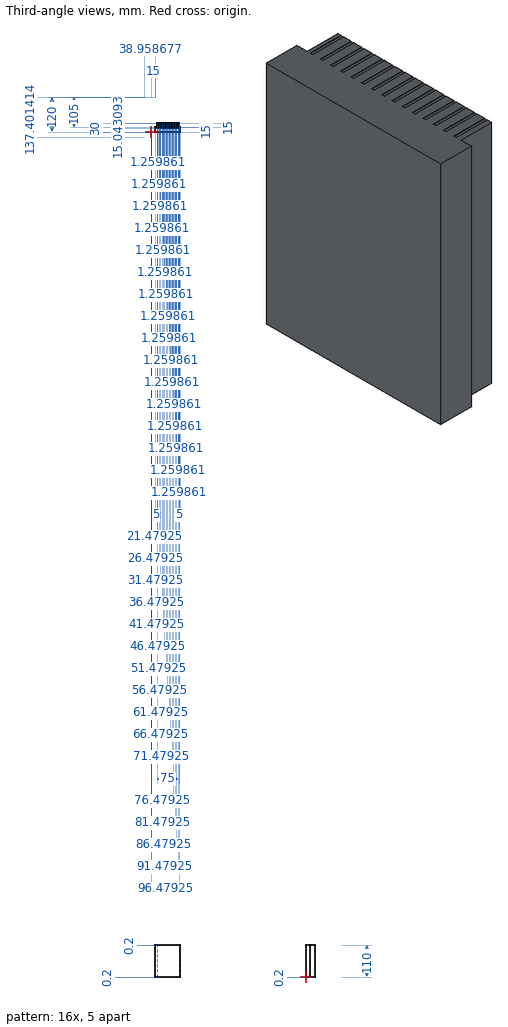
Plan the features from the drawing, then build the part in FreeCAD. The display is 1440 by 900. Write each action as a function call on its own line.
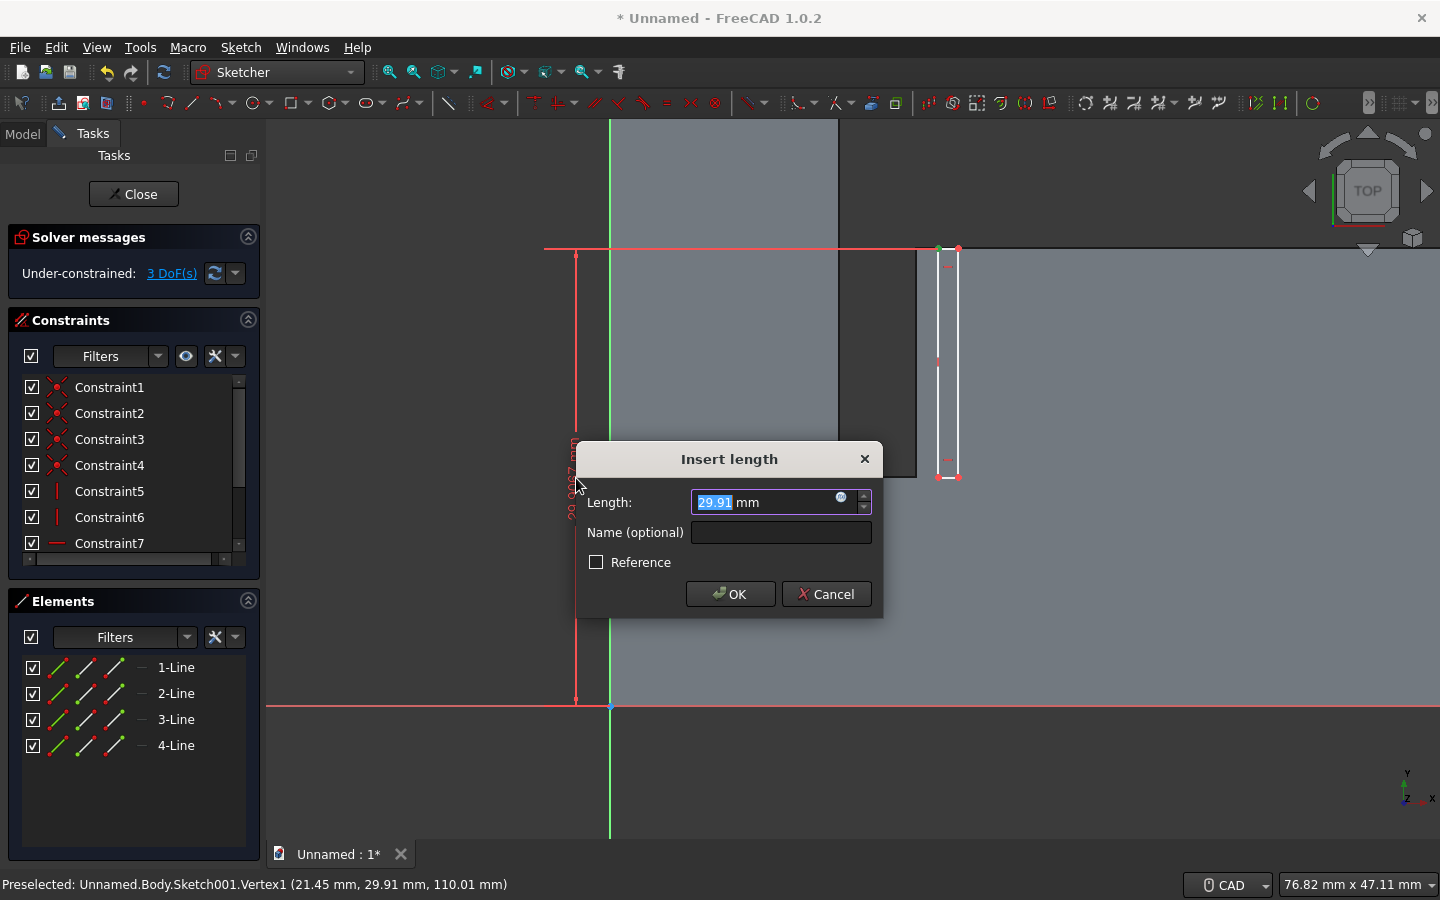
text(30)
key(Return)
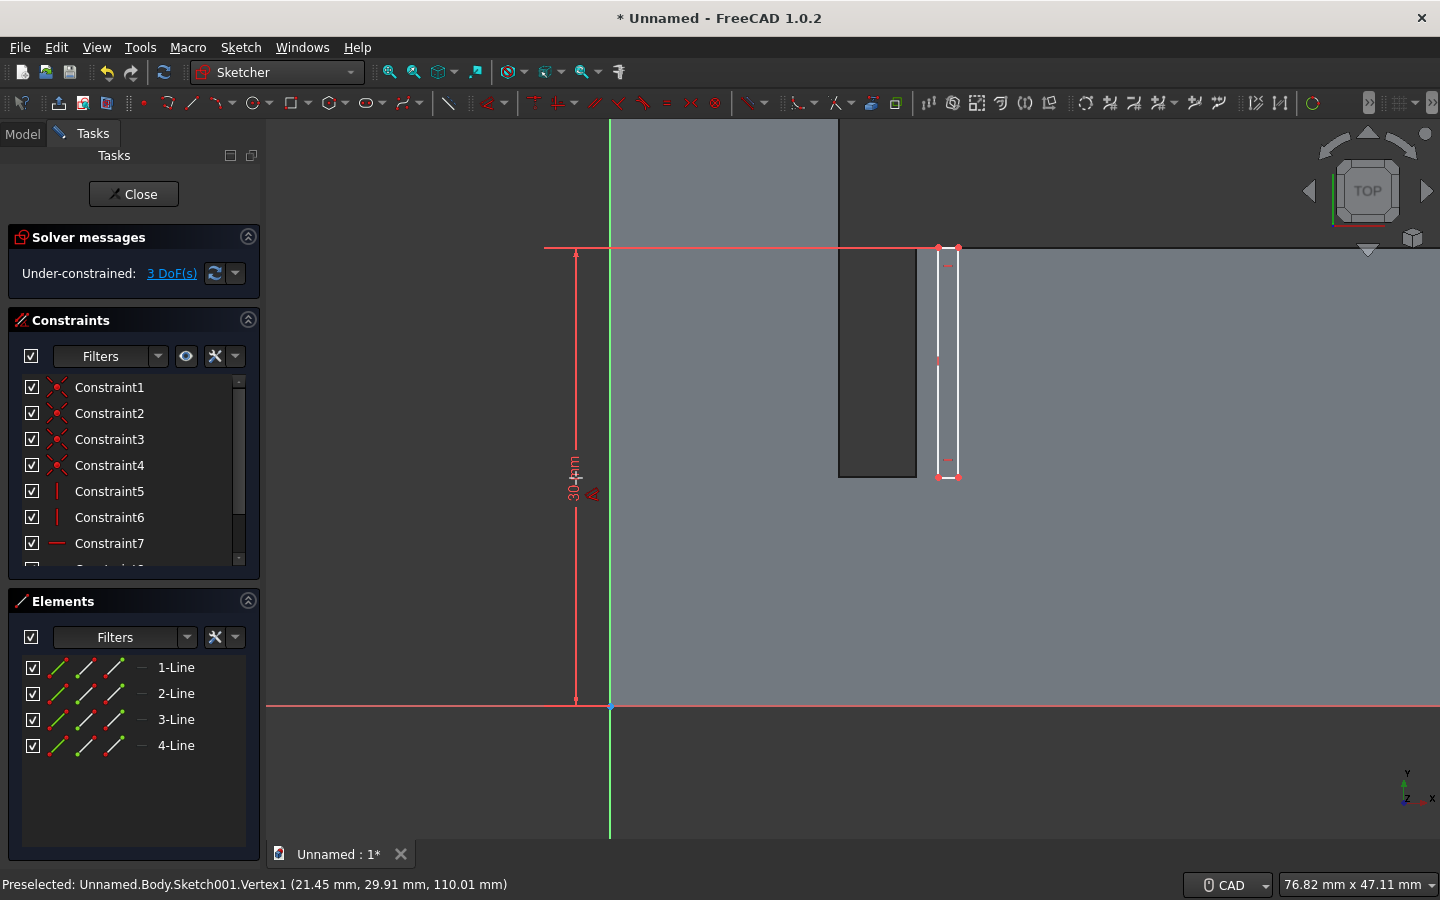
scroll(948, 478, up, 4)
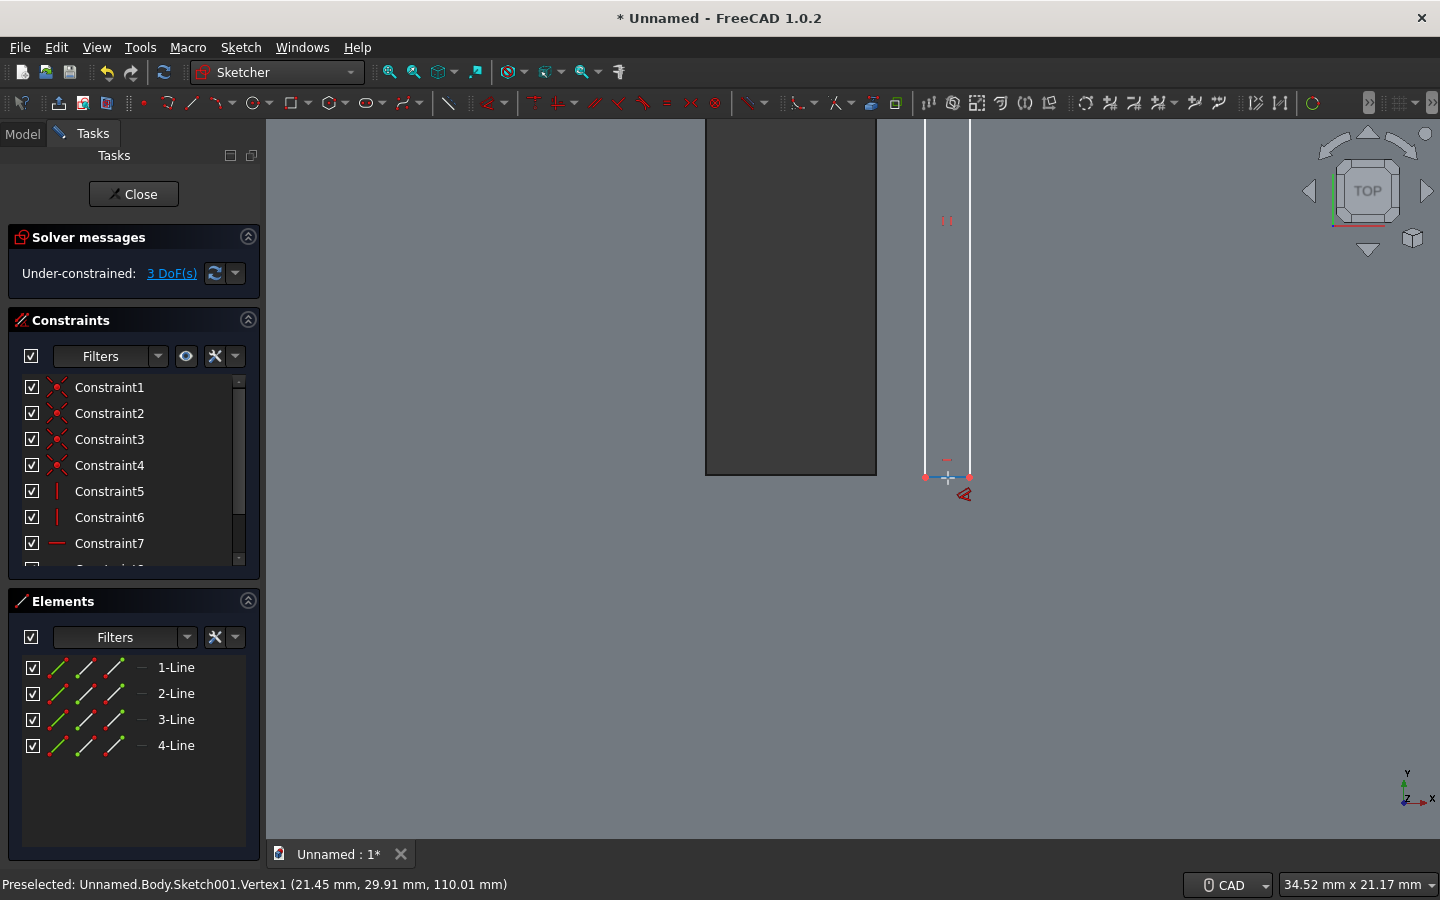
click(947, 477)
click(947, 511)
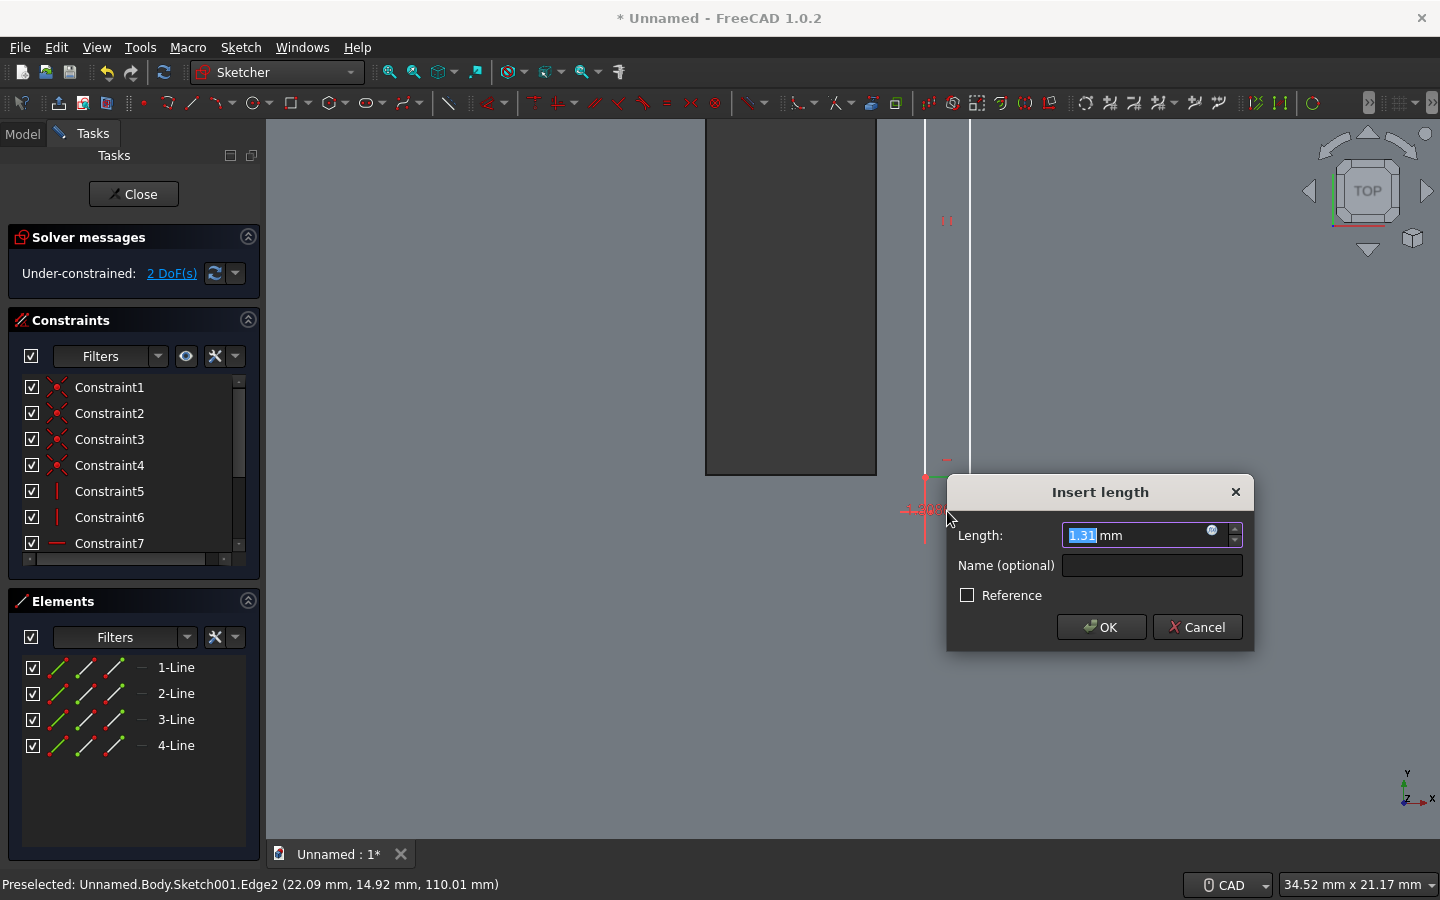
text(1.259861)
key(Return)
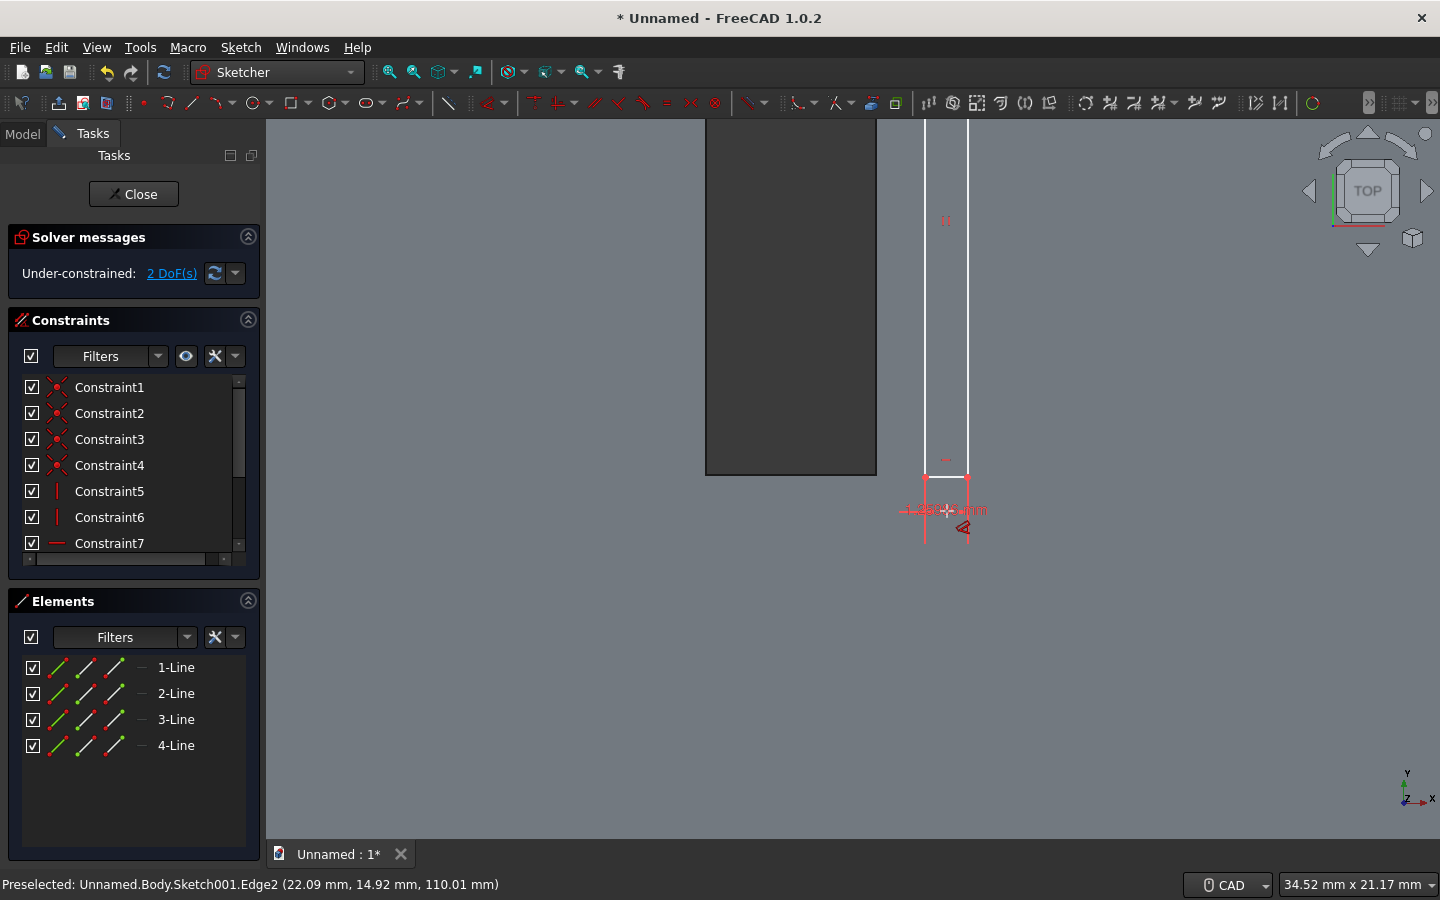
click(925, 324)
click(891, 312)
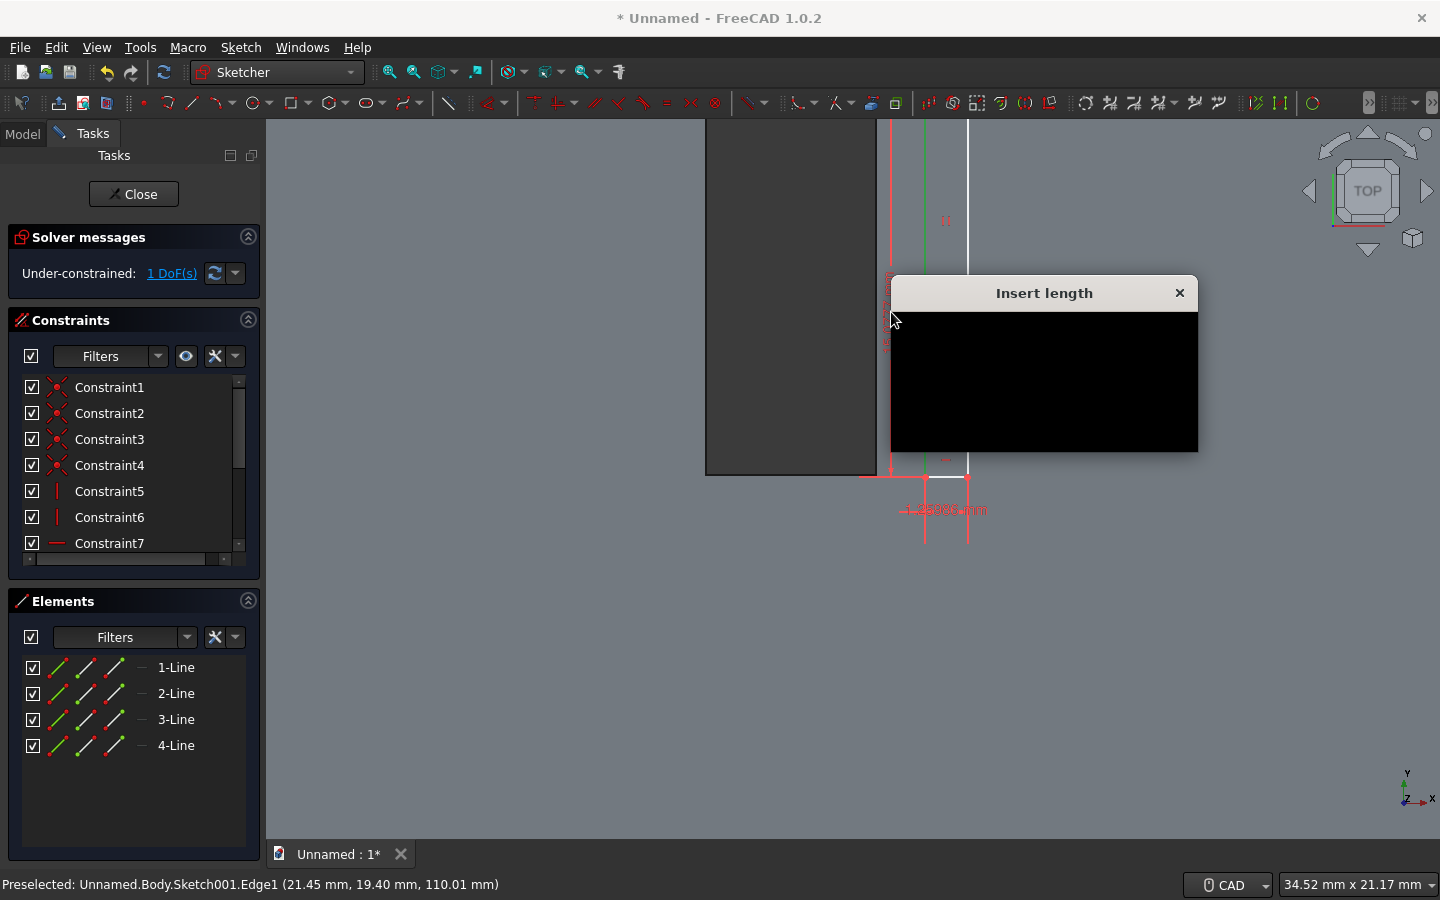
text(15.043093)
key(Return)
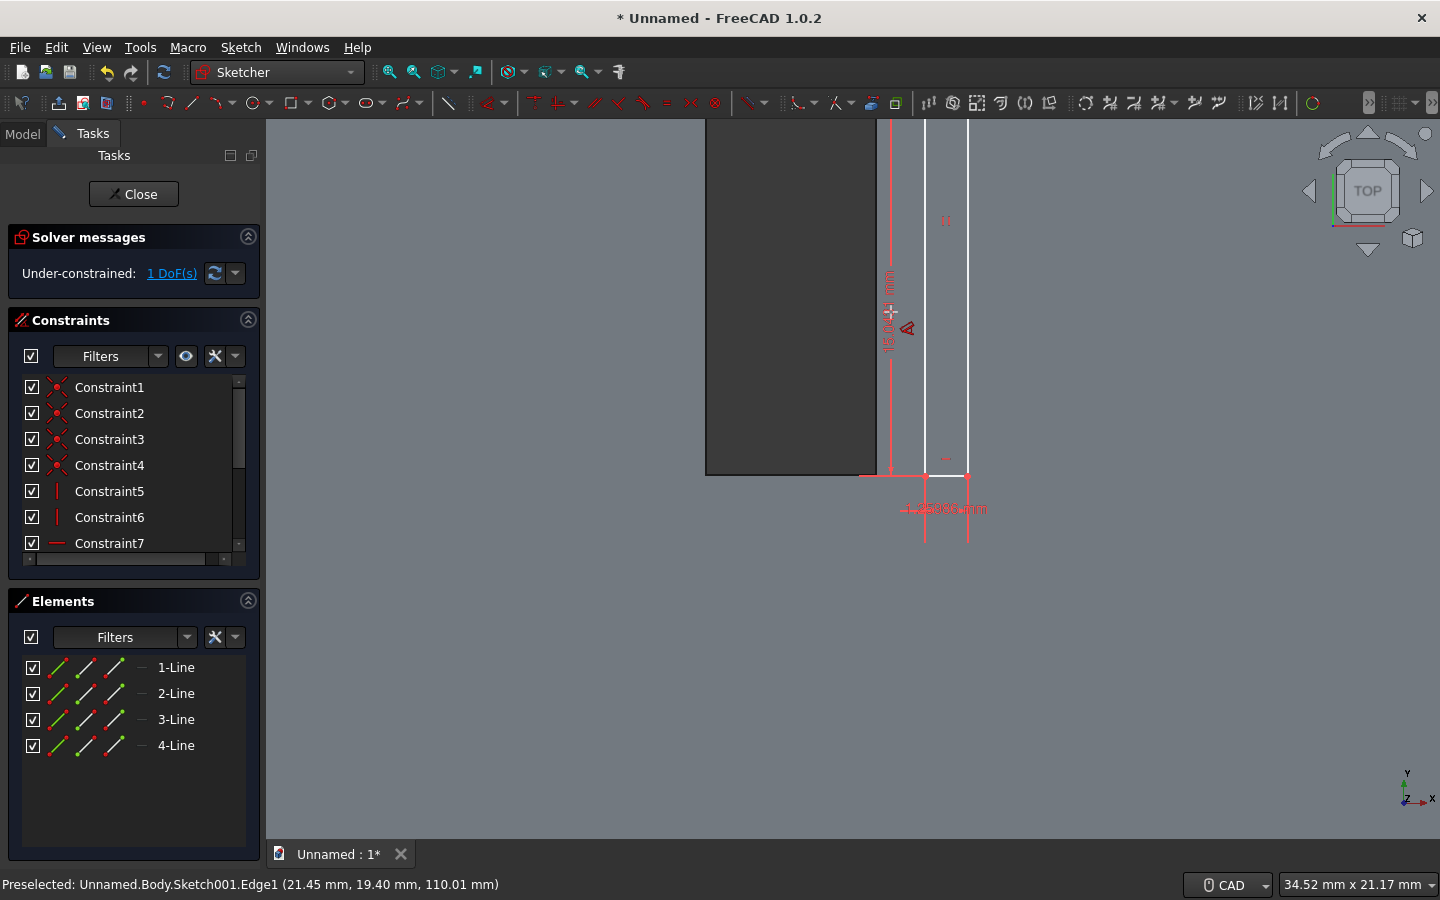
scroll(950, 482, down, 4)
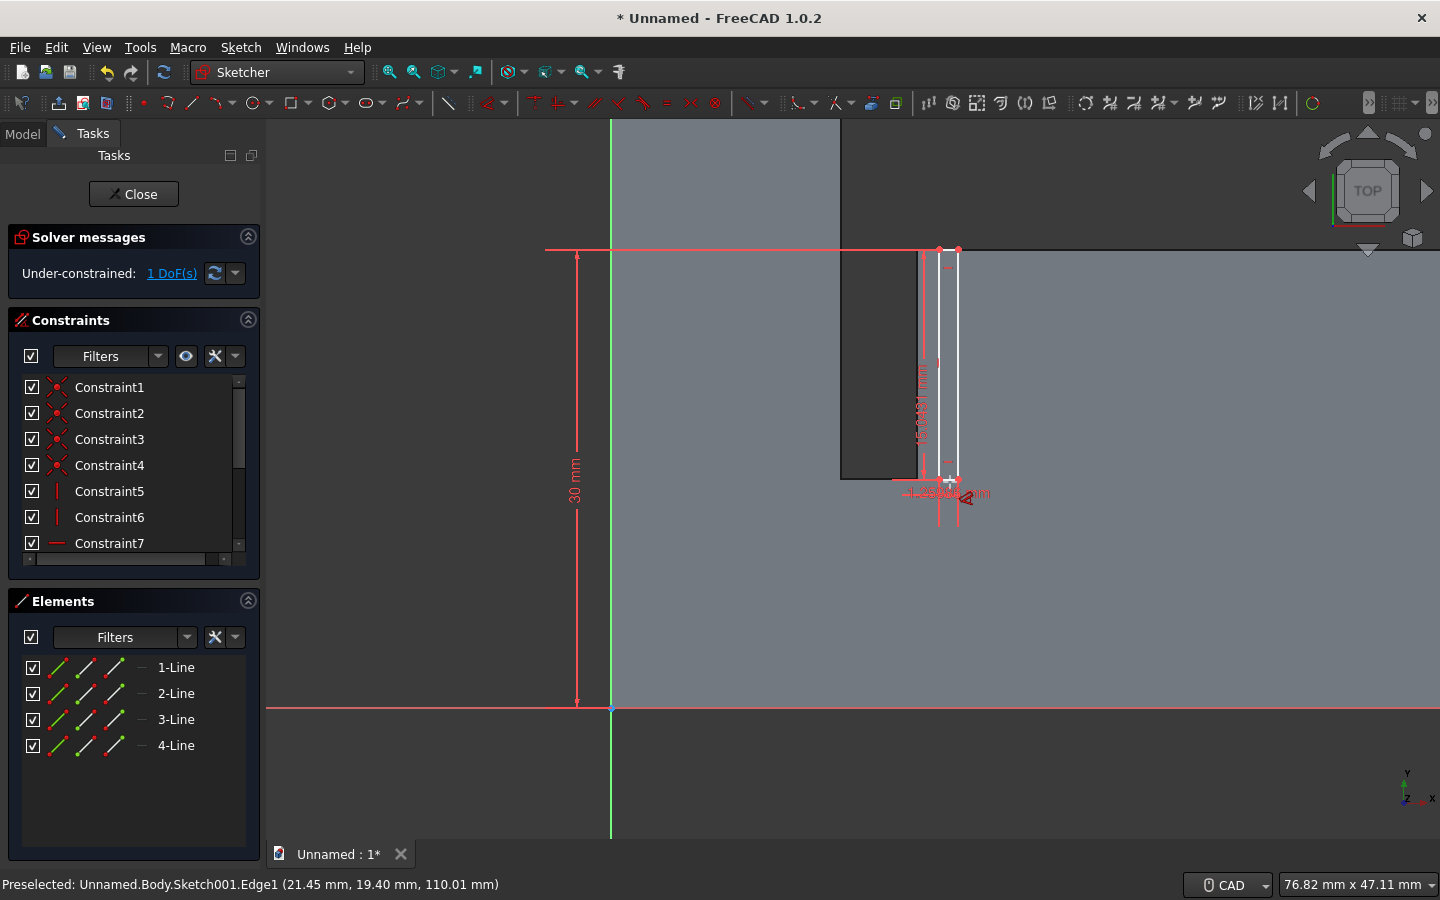
click(939, 250)
click(775, 742)